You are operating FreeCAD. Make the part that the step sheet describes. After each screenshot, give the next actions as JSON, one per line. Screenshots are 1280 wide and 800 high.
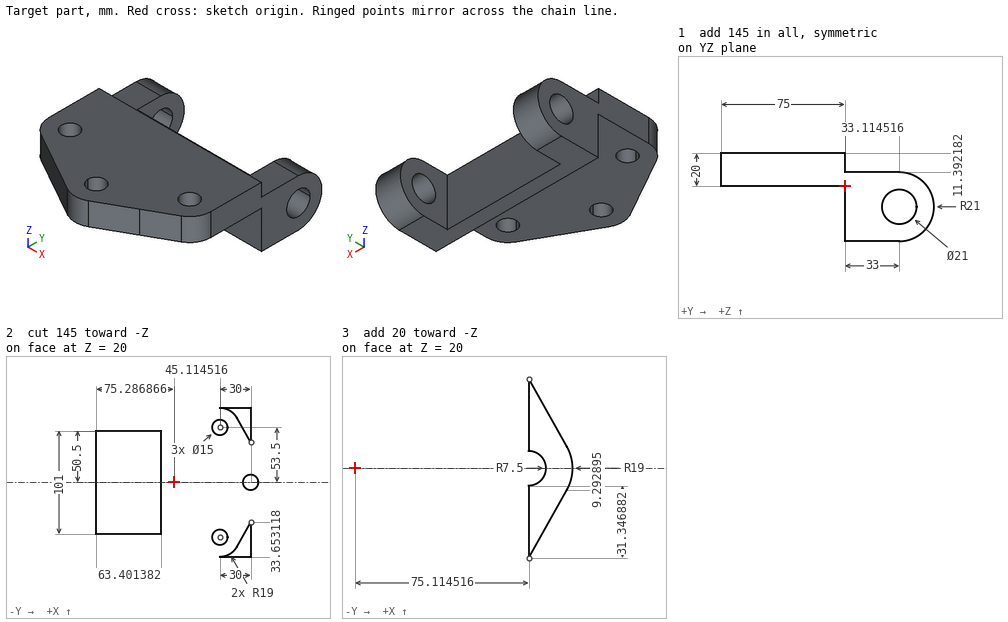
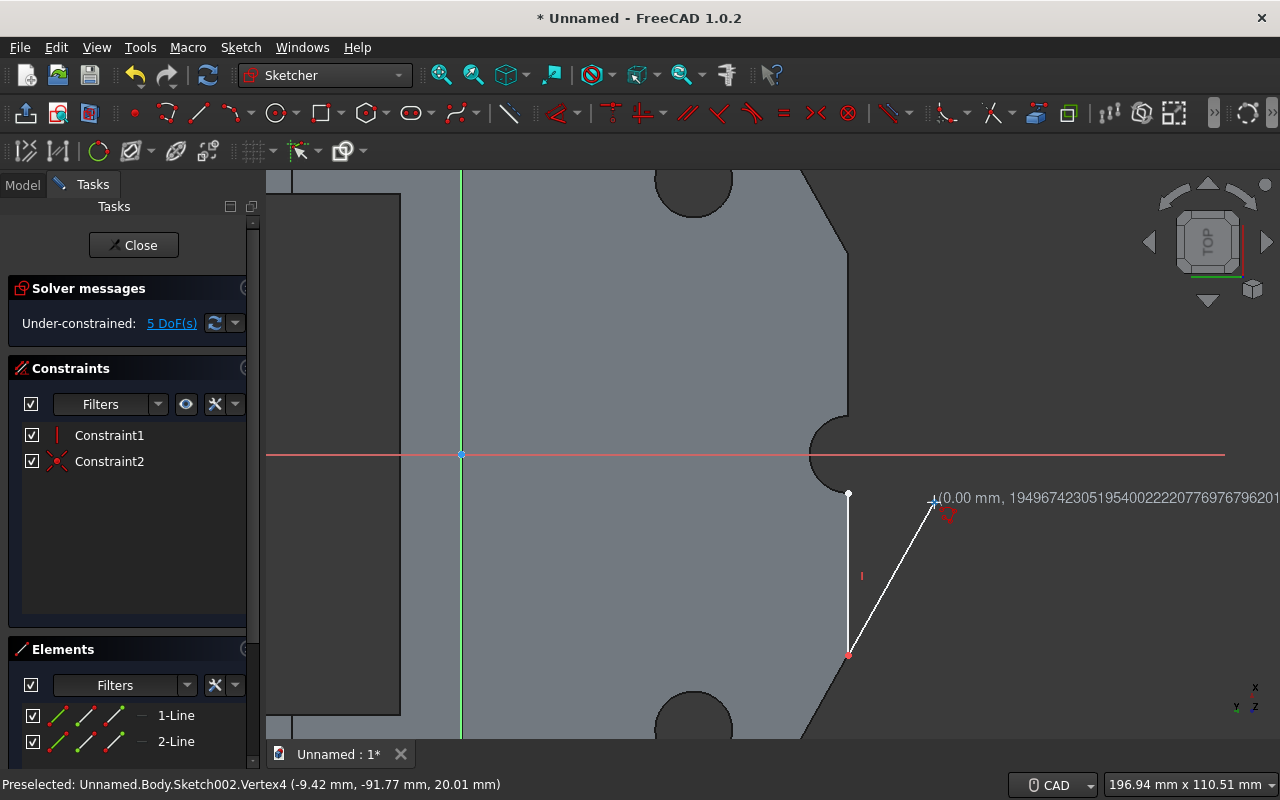
{"action": "left_click", "coordinate": [934, 407]}
{"action": "left_click", "coordinate": [848, 254]}
{"action": "left_click", "coordinate": [848, 416]}
{"action": "right_click", "coordinate": [848, 416]}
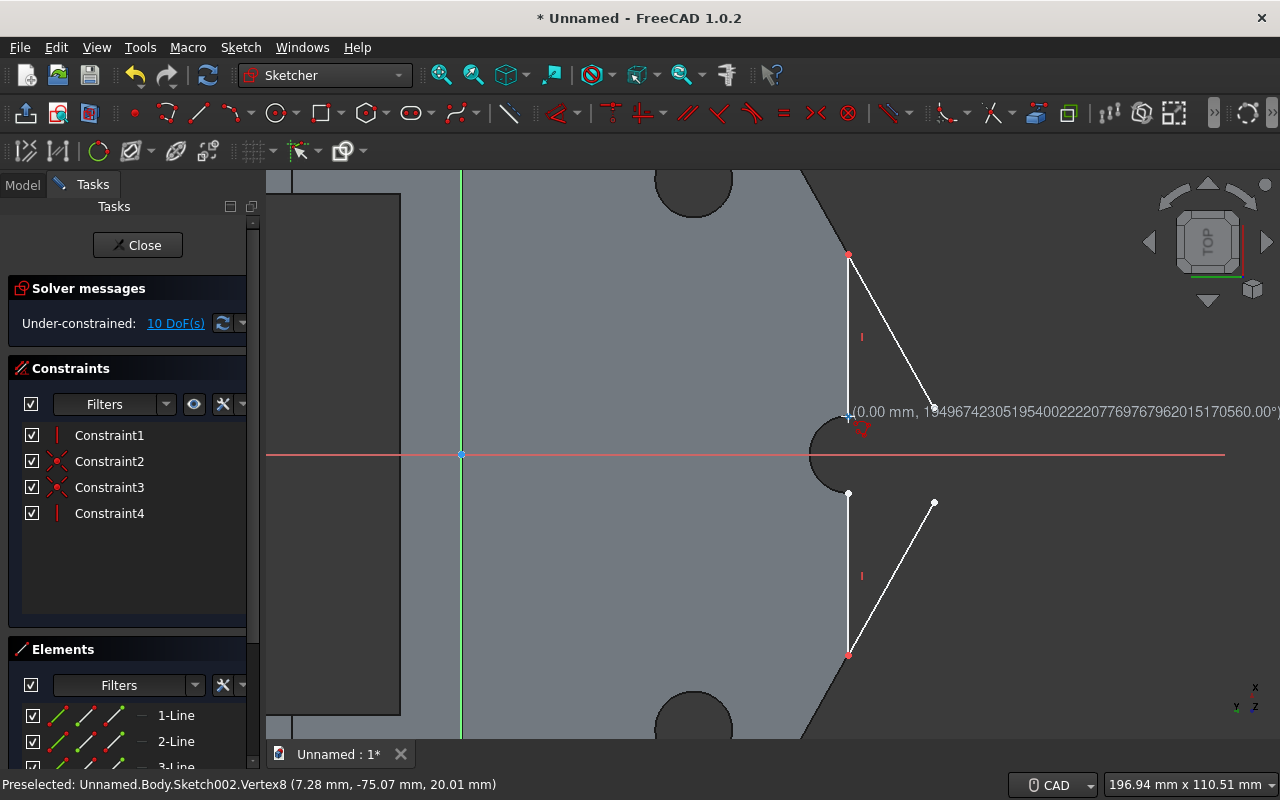
{"action": "left_click", "coordinate": [232, 114]}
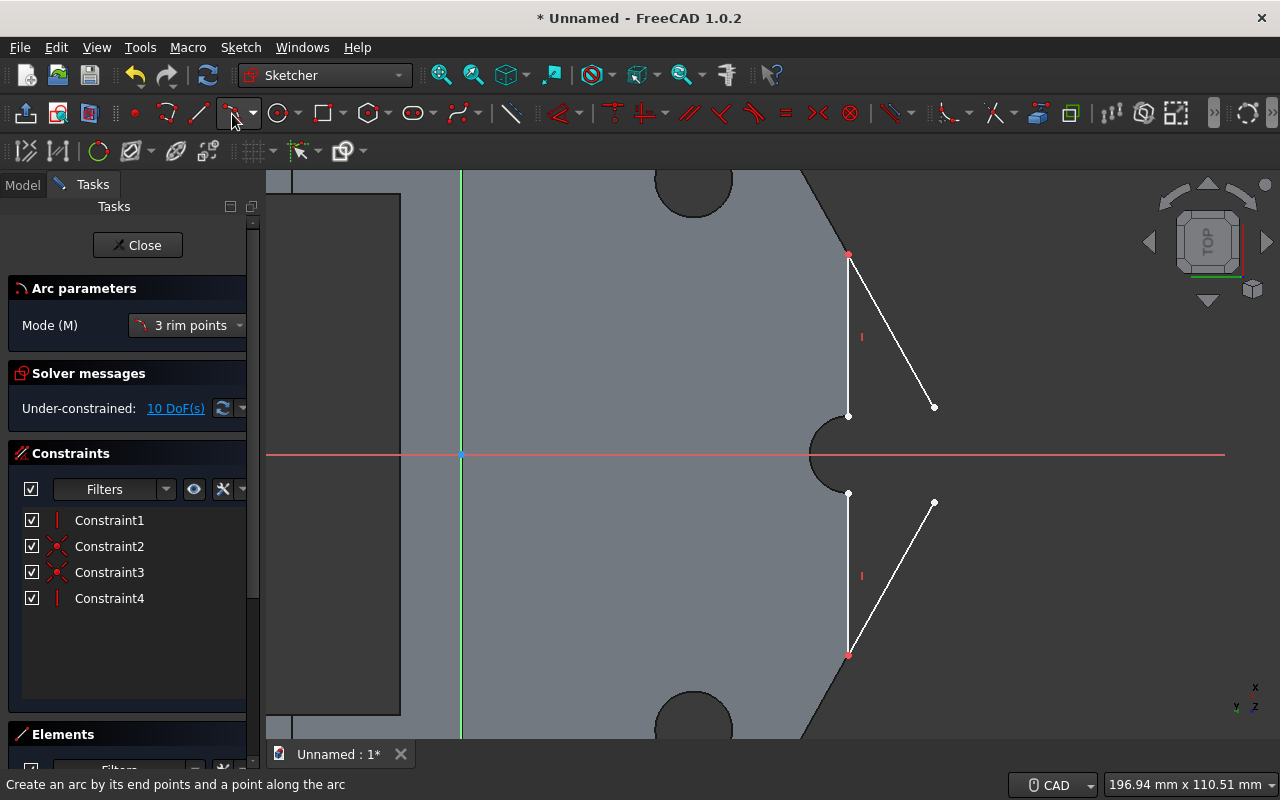
{"action": "left_click", "coordinate": [934, 503]}
{"action": "left_click", "coordinate": [934, 408]}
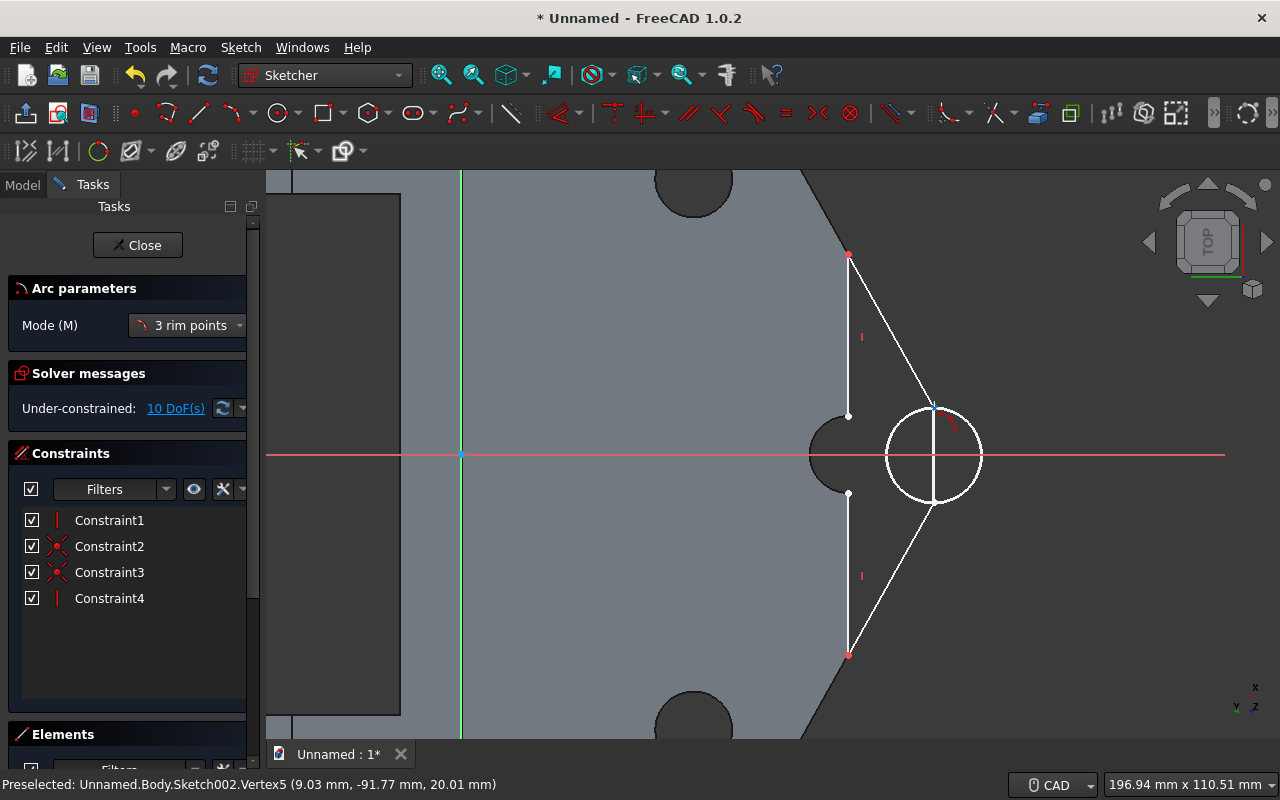
{"action": "scroll", "coordinate": [944, 474], "scroll_direction": "up", "scroll_amount": 3}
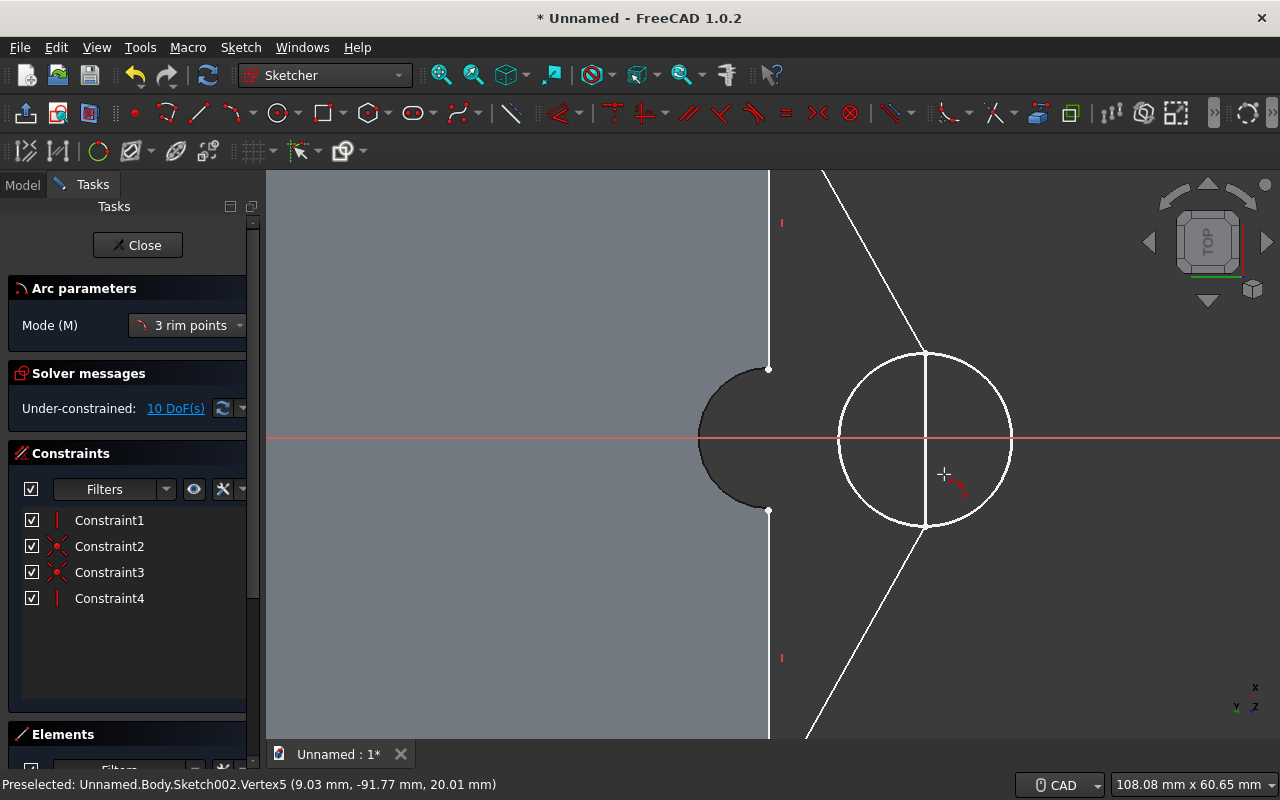
{"action": "left_click", "coordinate": [943, 474]}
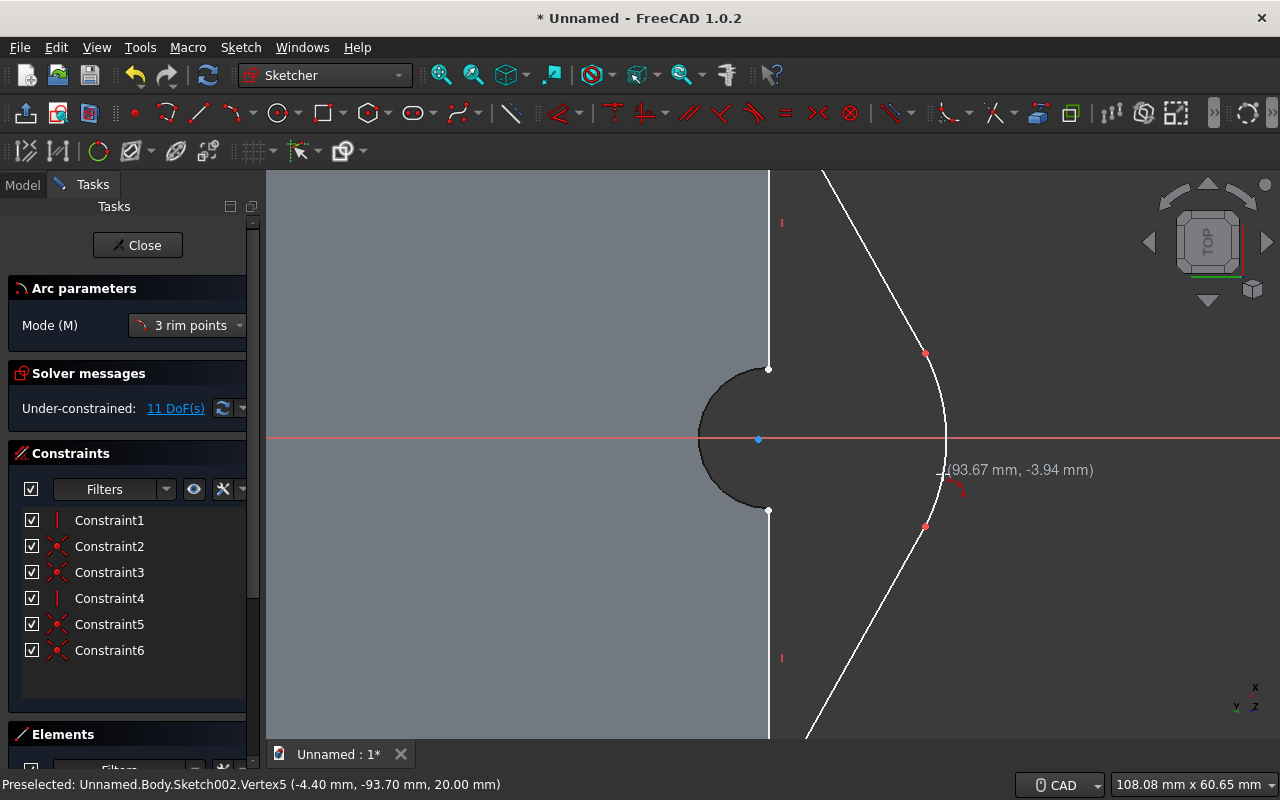
{"action": "left_click", "coordinate": [769, 370]}
{"action": "left_click", "coordinate": [769, 510]}
{"action": "left_click", "coordinate": [826, 479]}
{"action": "key", "text": "Escape"}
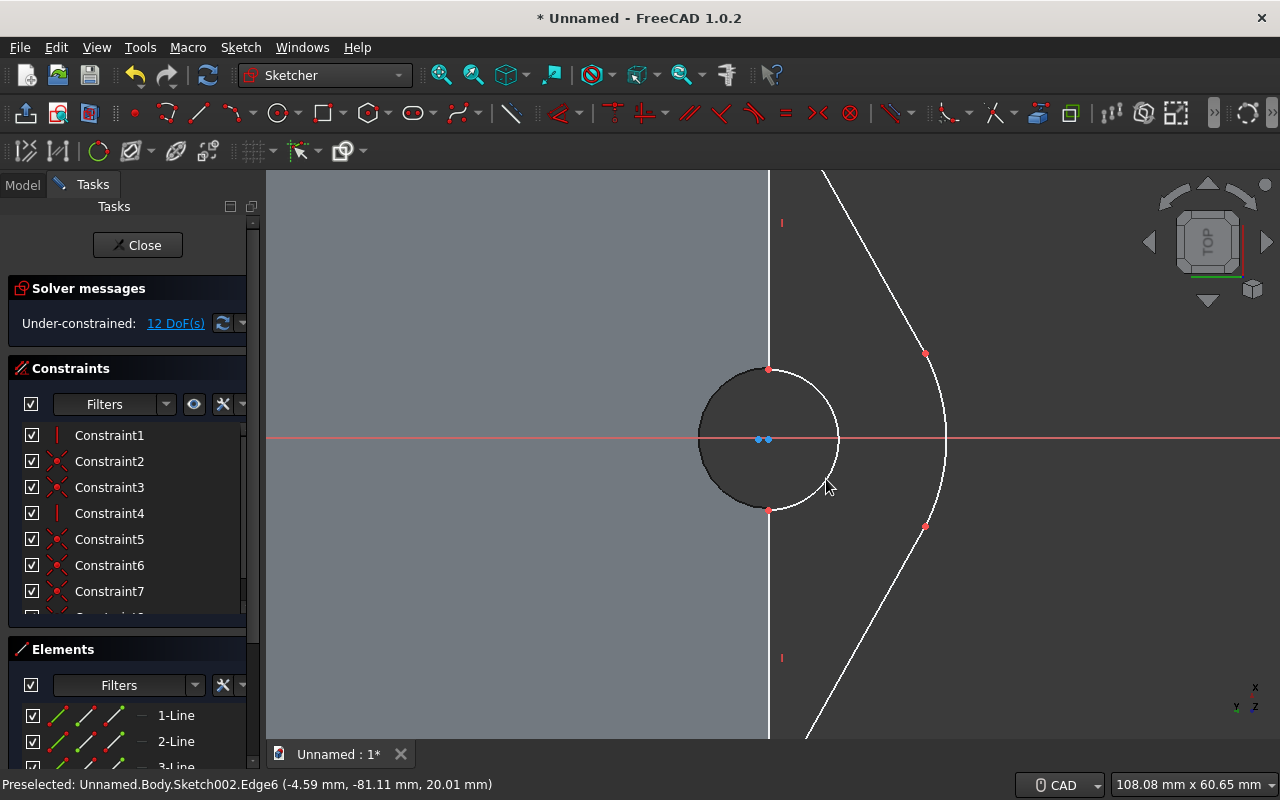
{"action": "left_click", "coordinate": [878, 610]}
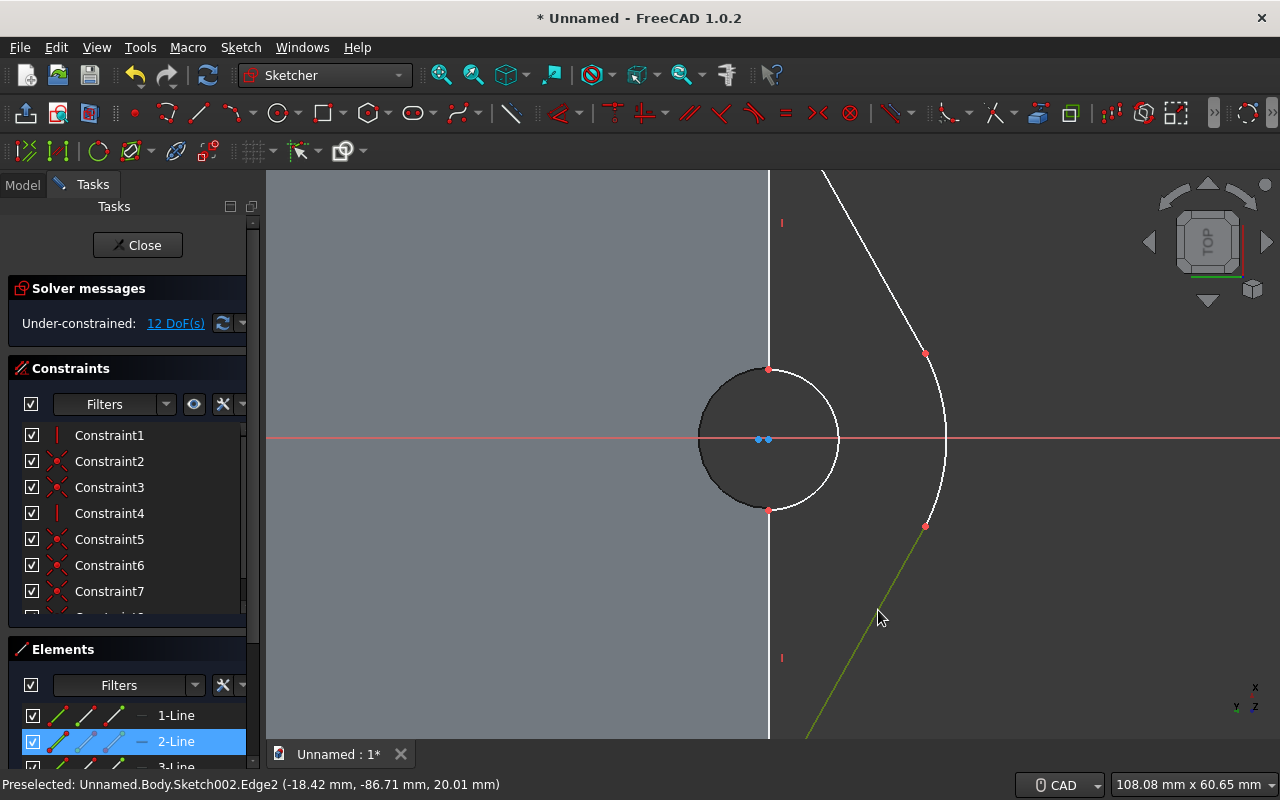
{"action": "left_click", "coordinate": [943, 476]}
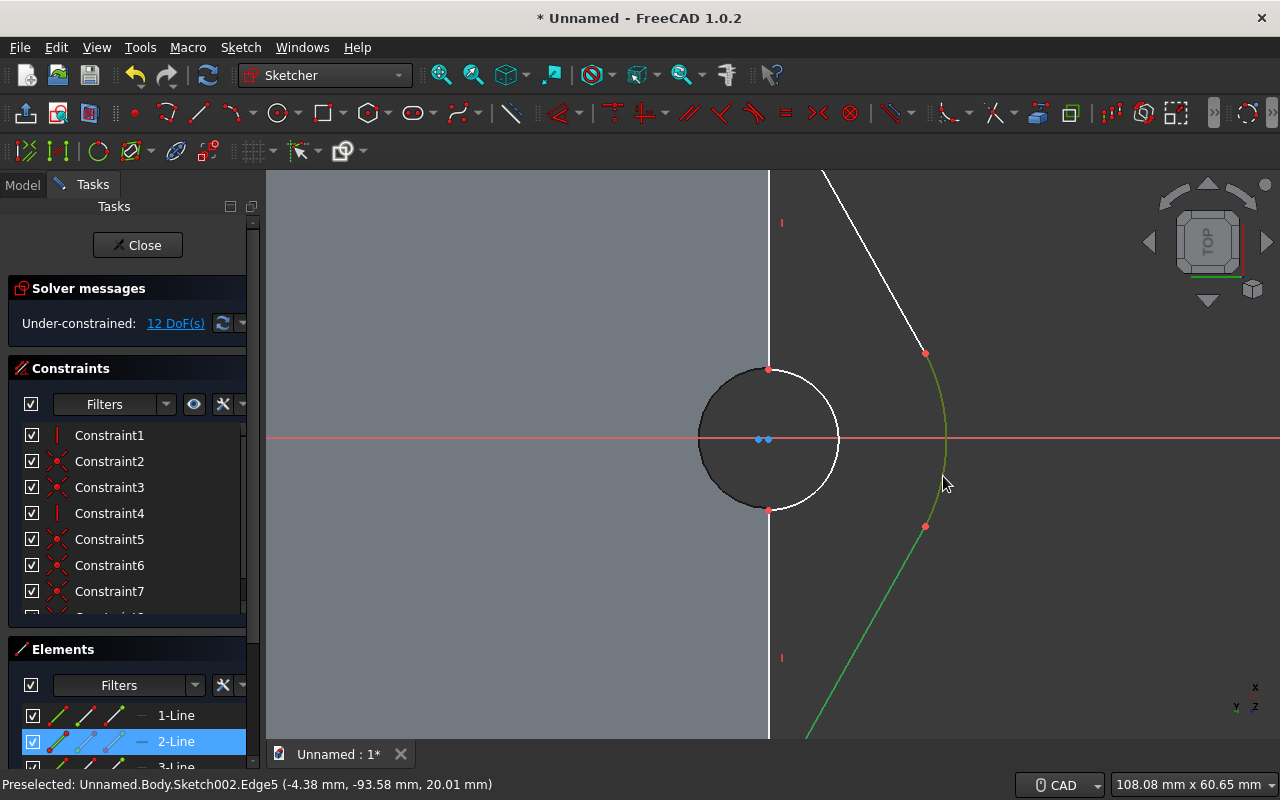
{"action": "left_click", "coordinate": [754, 114]}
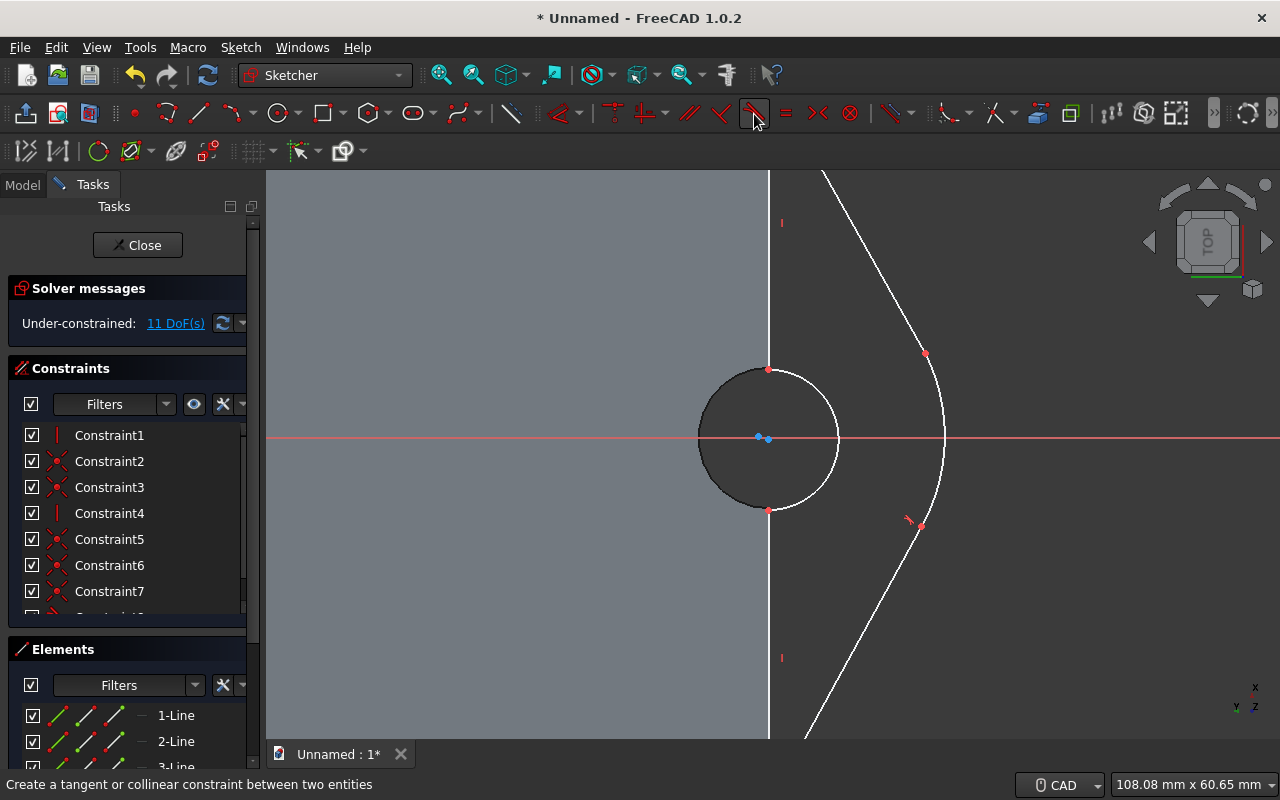
{"action": "left_click", "coordinate": [878, 270]}